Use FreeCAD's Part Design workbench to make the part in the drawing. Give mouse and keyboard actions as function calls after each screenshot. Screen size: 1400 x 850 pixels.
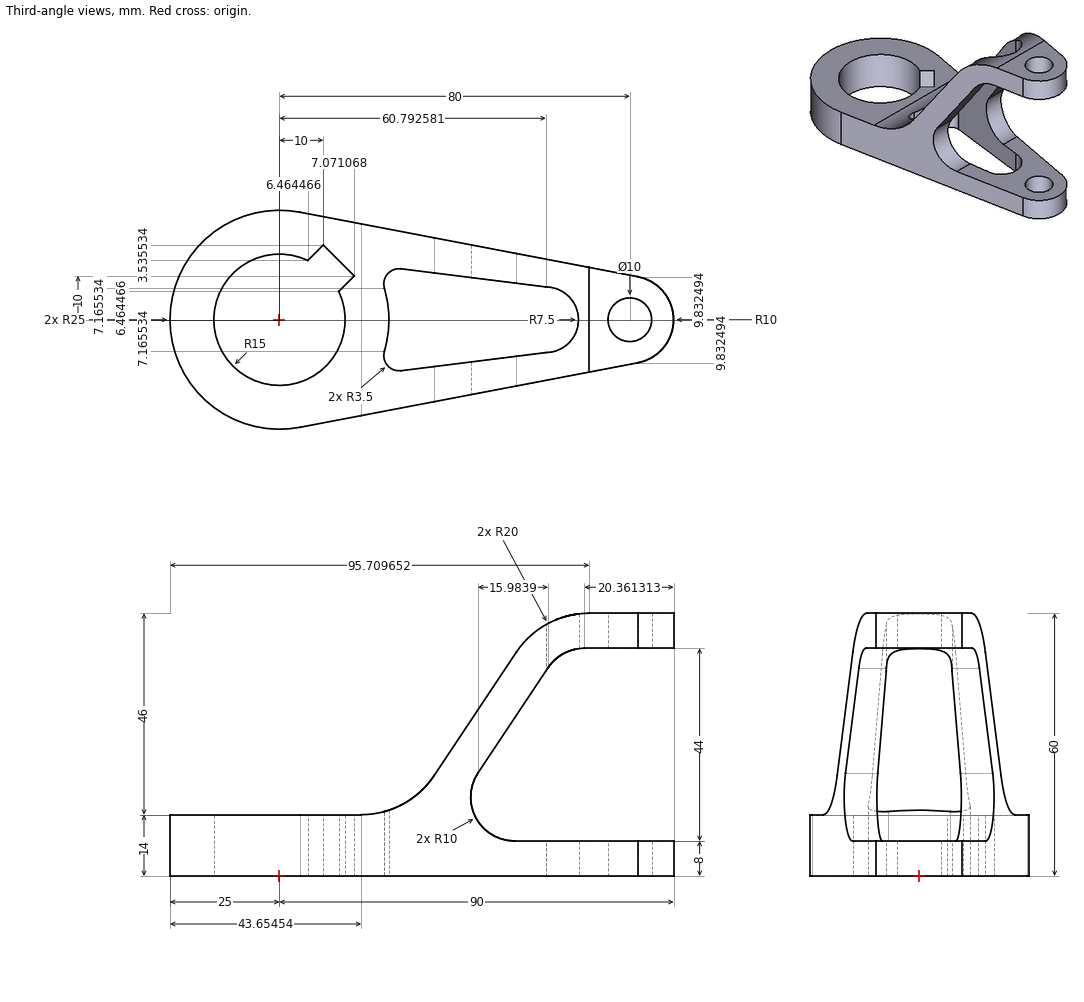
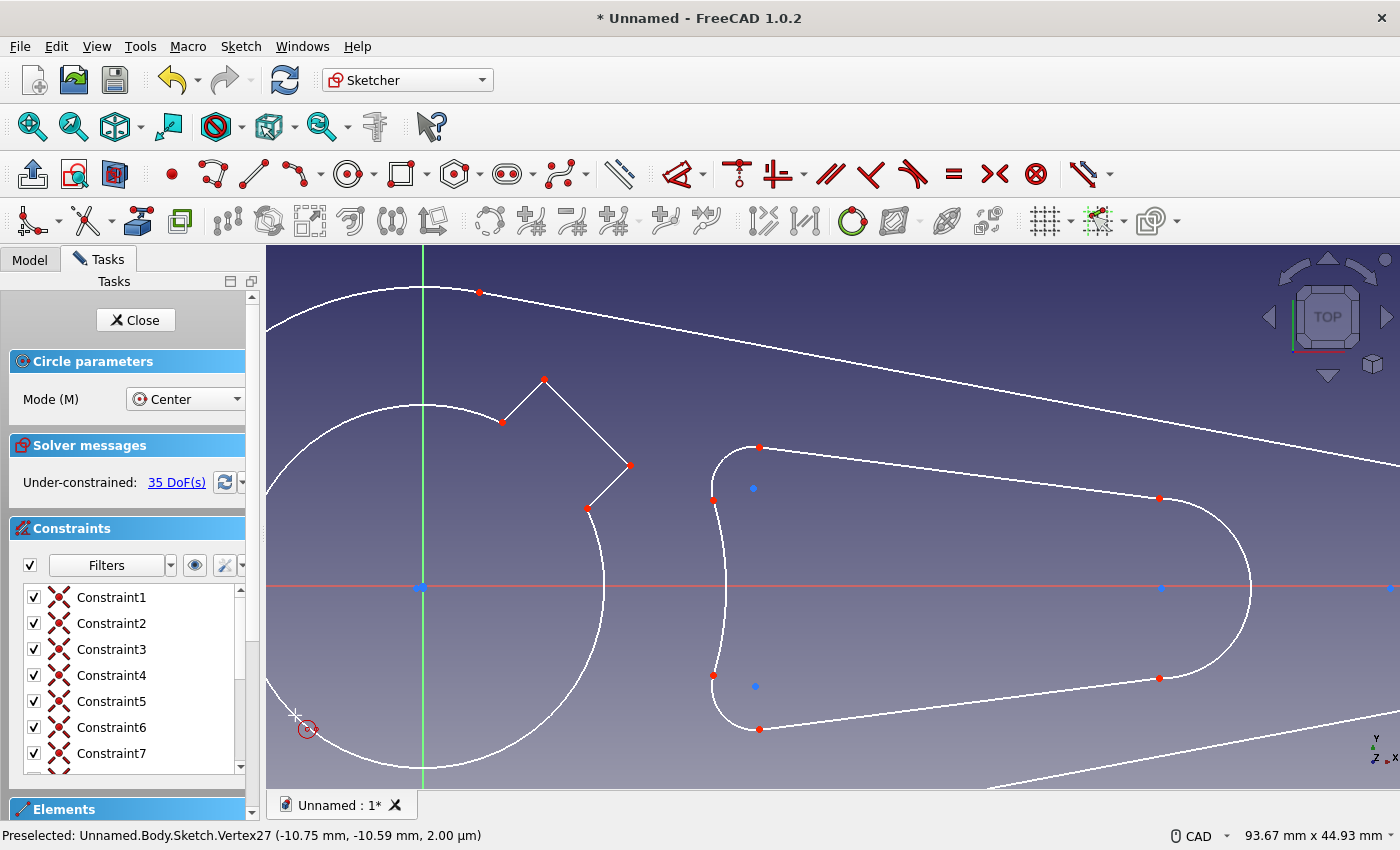
scroll(722, 461, down, 4)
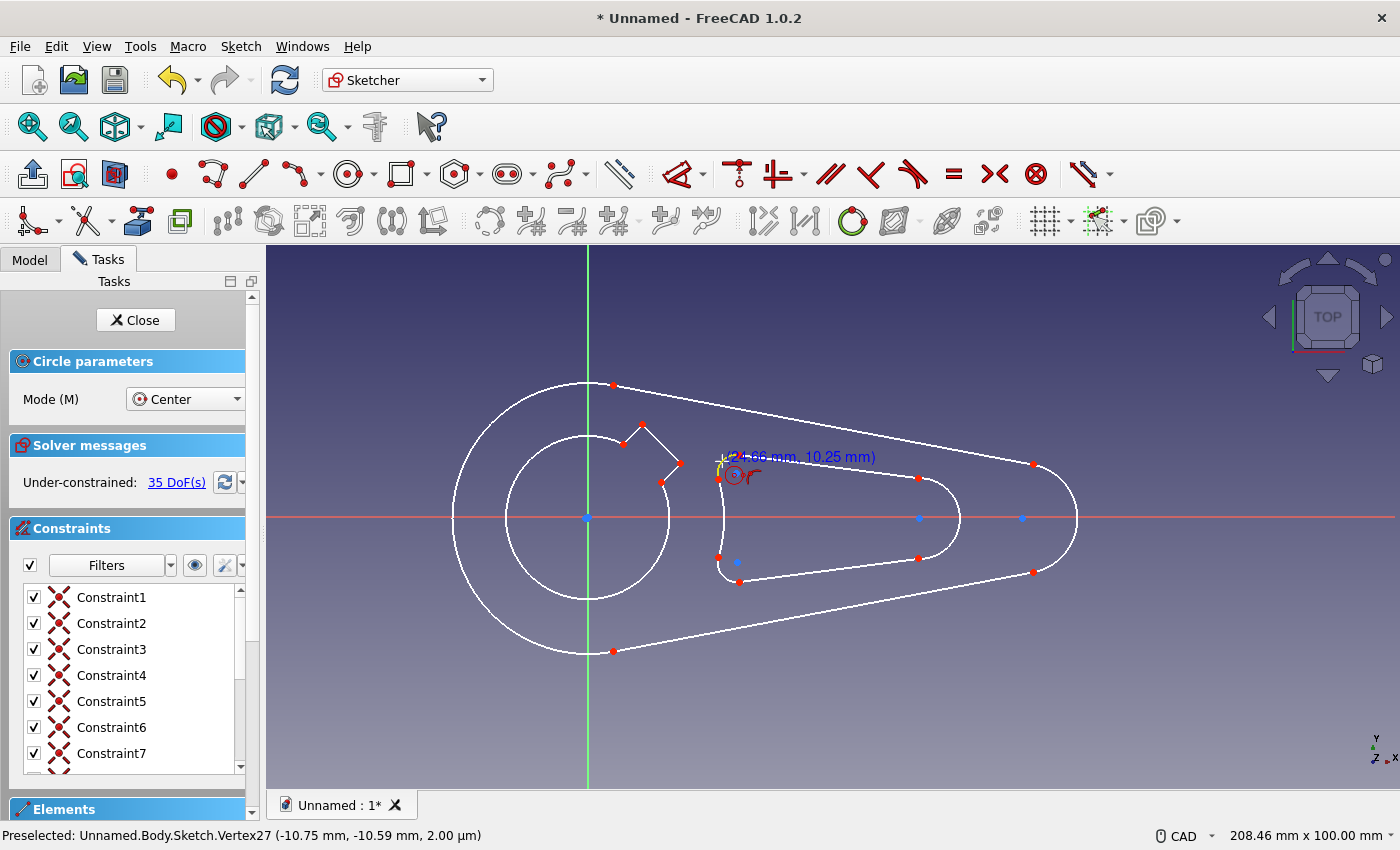
click(1023, 517)
move(1042, 498)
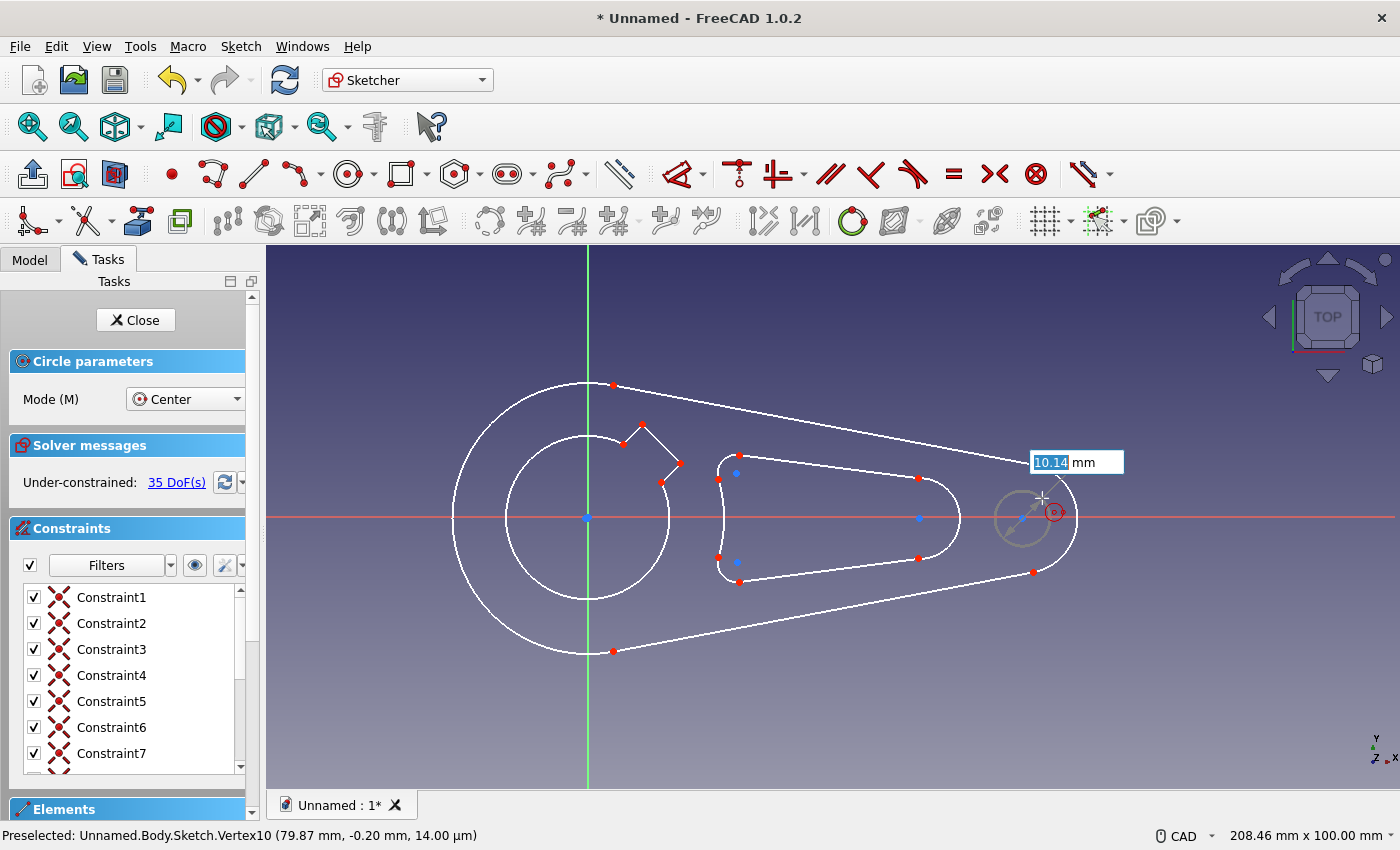
text(10)
key(Return)
key(Escape)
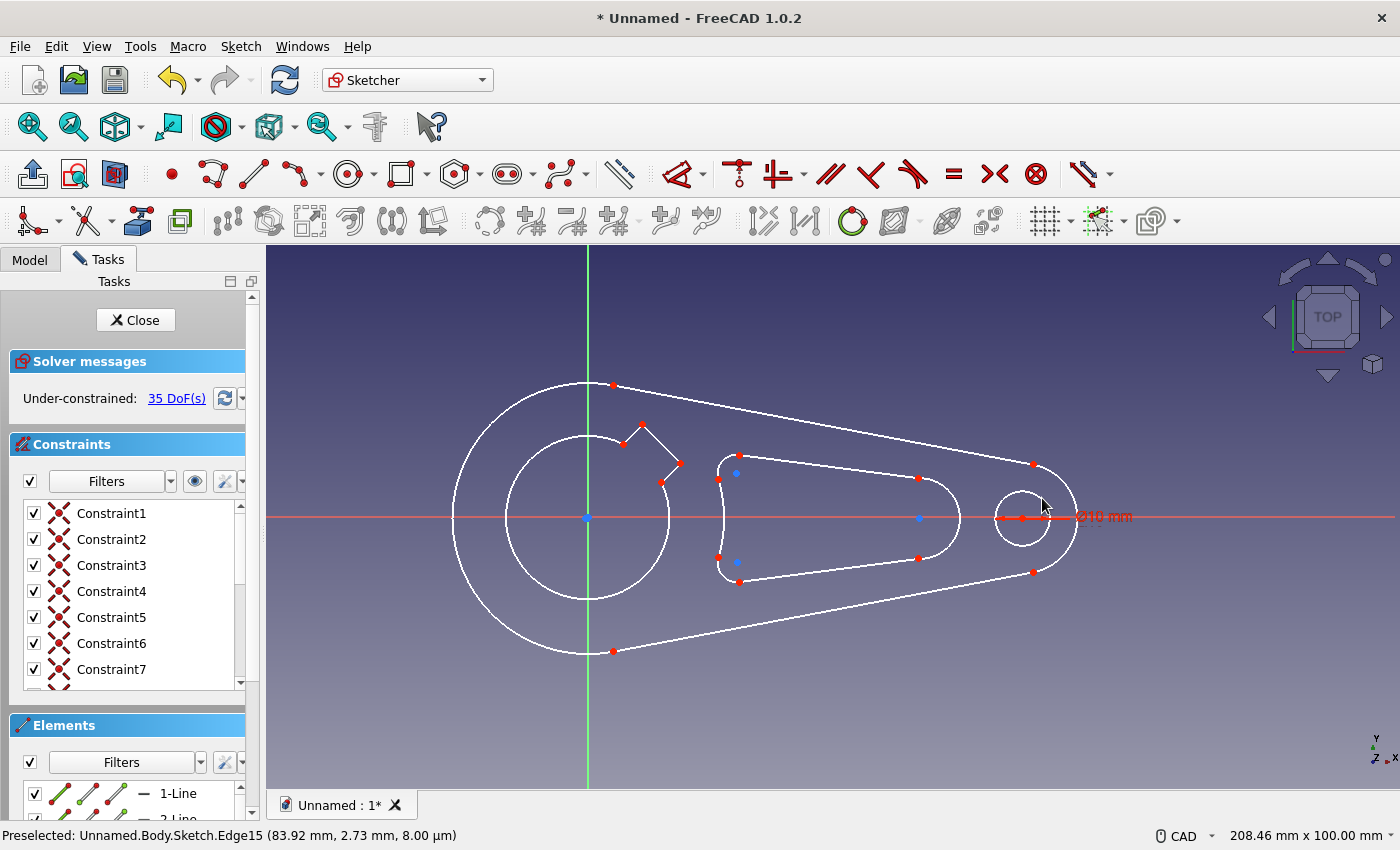
click(907, 441)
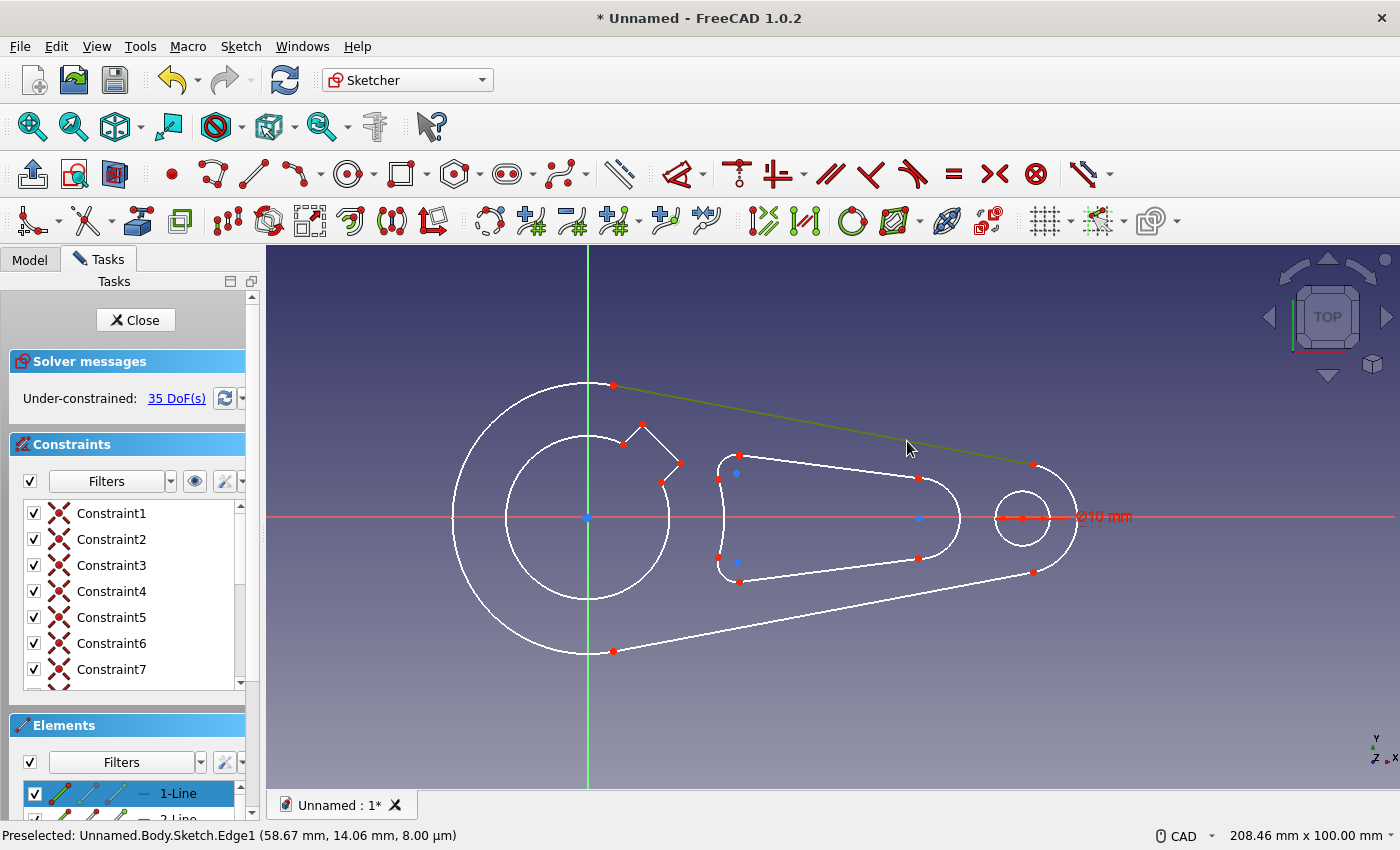
click(485, 431)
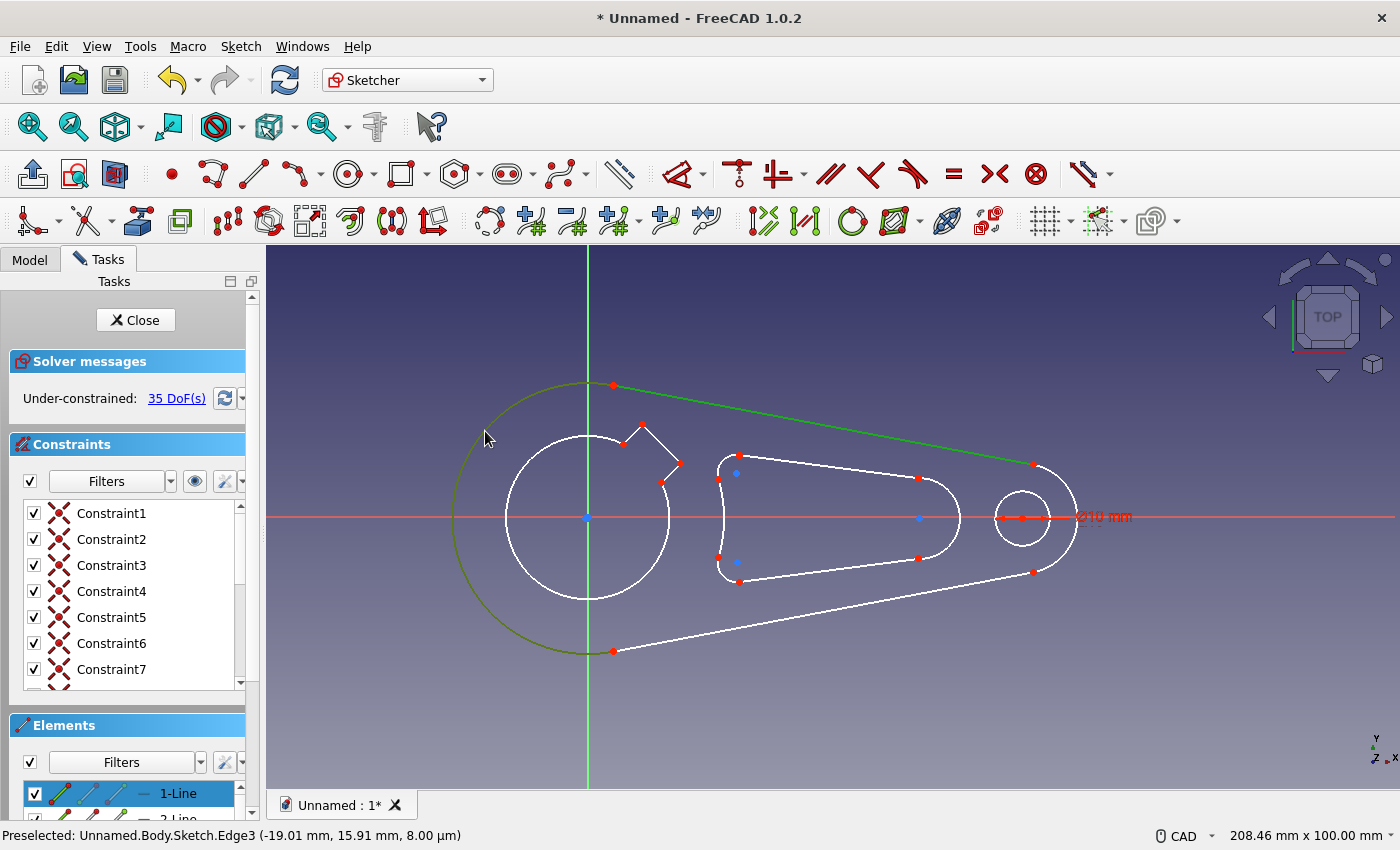
click(913, 174)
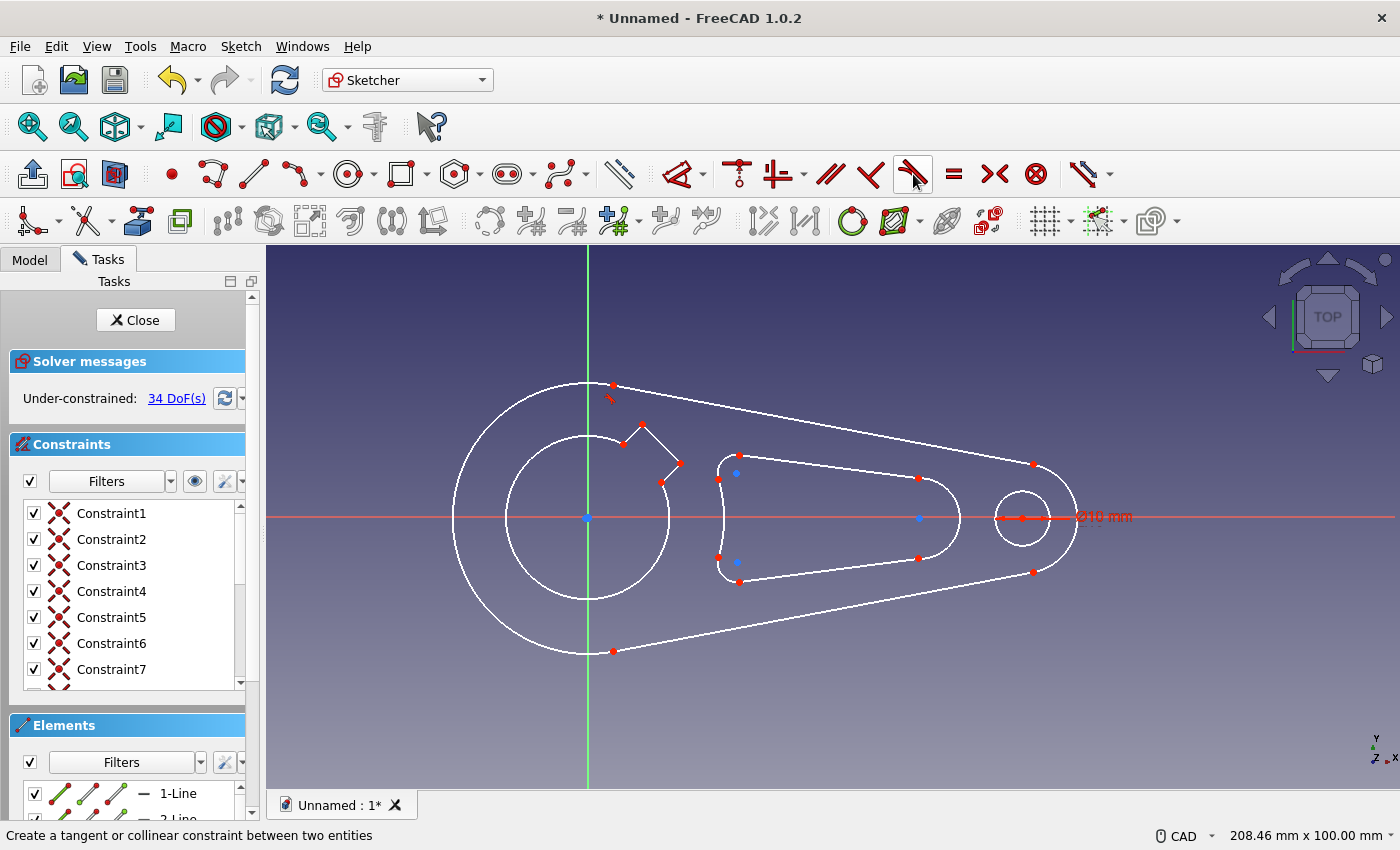
click(739, 628)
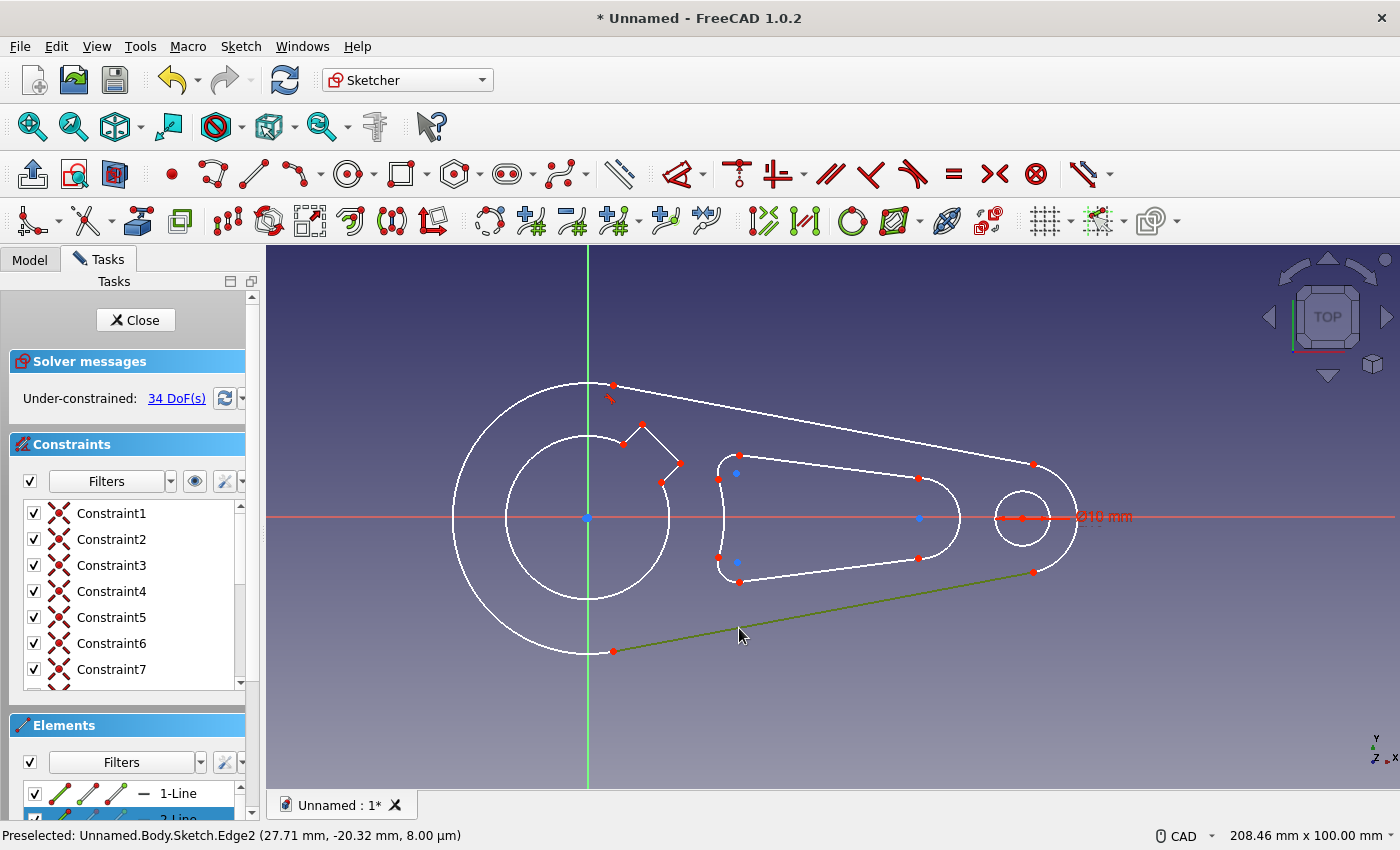
click(485, 431)